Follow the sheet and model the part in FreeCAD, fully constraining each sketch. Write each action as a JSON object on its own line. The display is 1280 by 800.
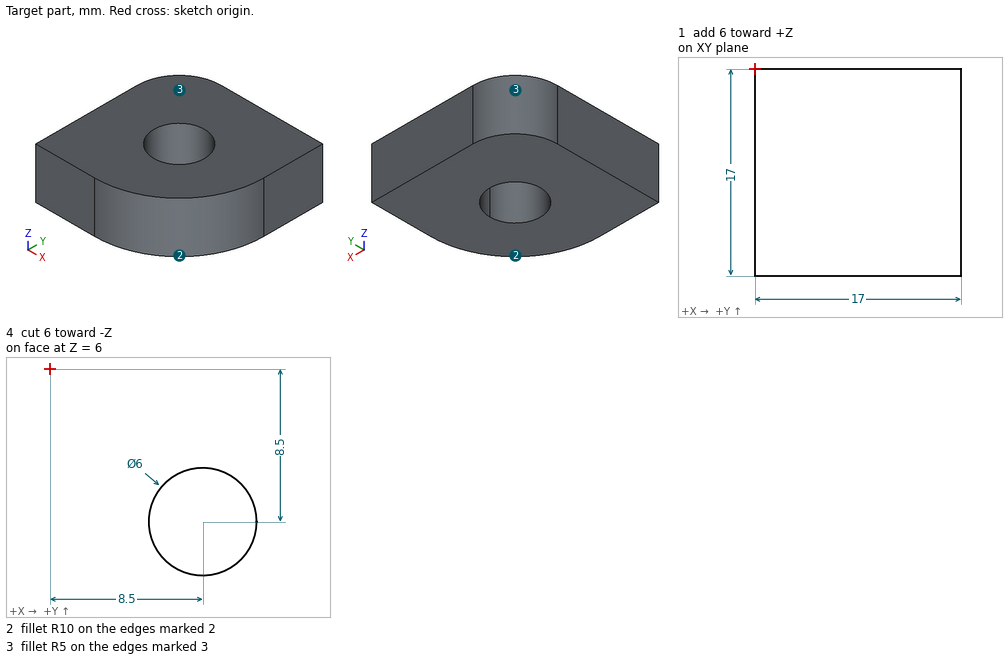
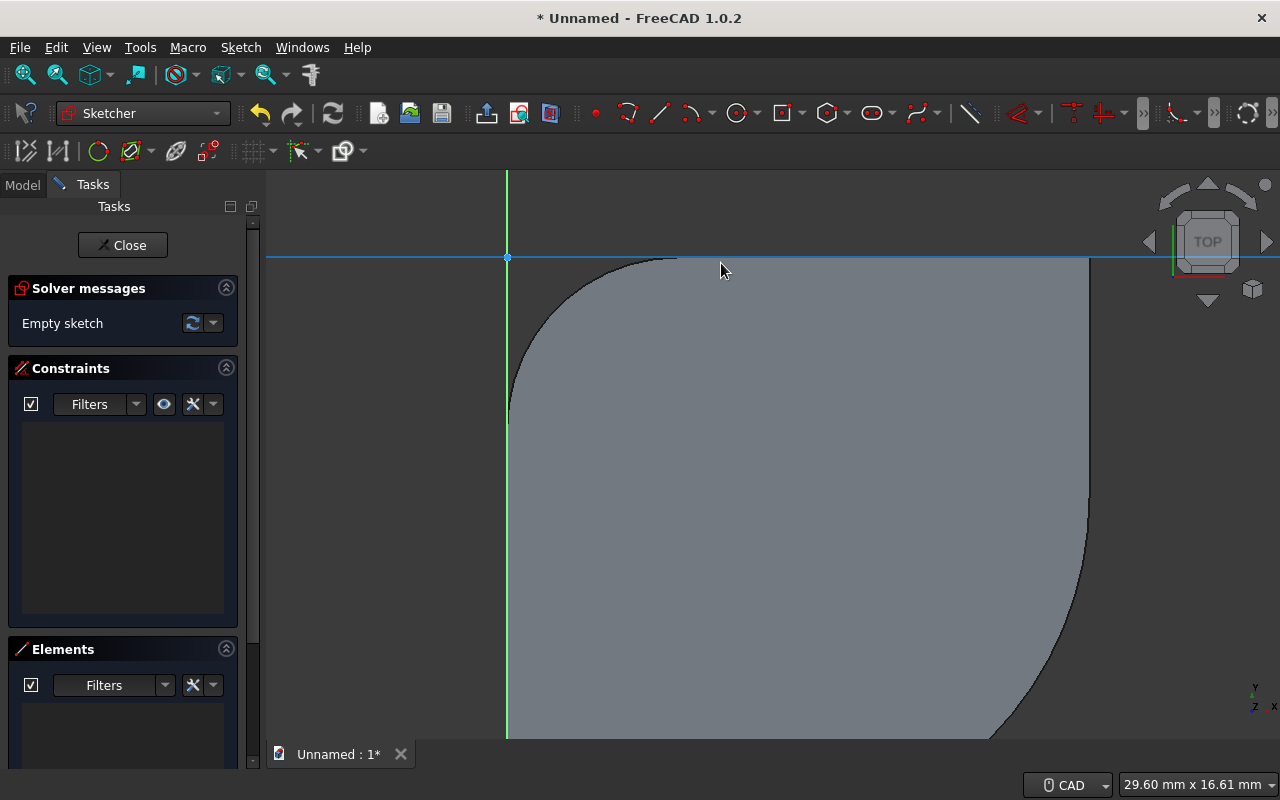
{"action": "left_click", "coordinate": [738, 114]}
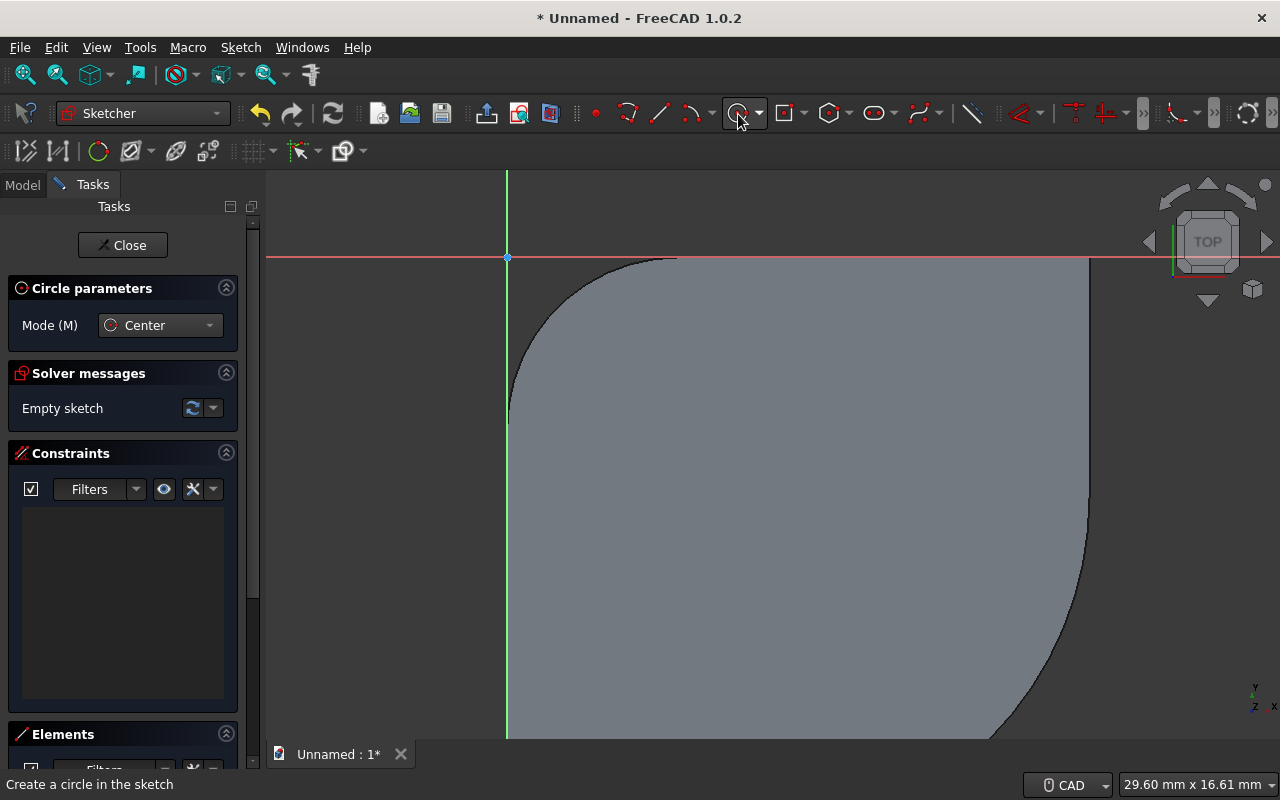
{"action": "left_click", "coordinate": [798, 549]}
{"action": "left_click", "coordinate": [871, 476]}
{"action": "key", "text": "Escape"}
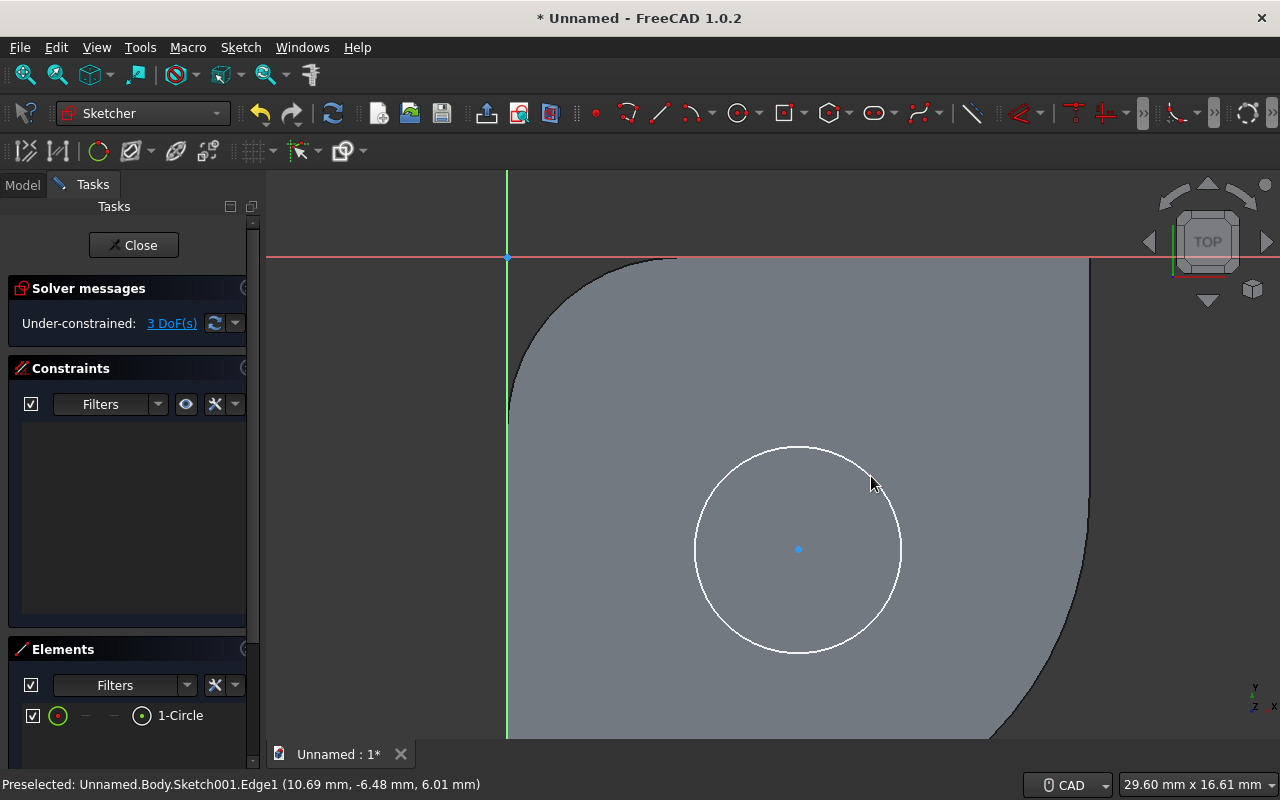
{"action": "left_click", "coordinate": [871, 477]}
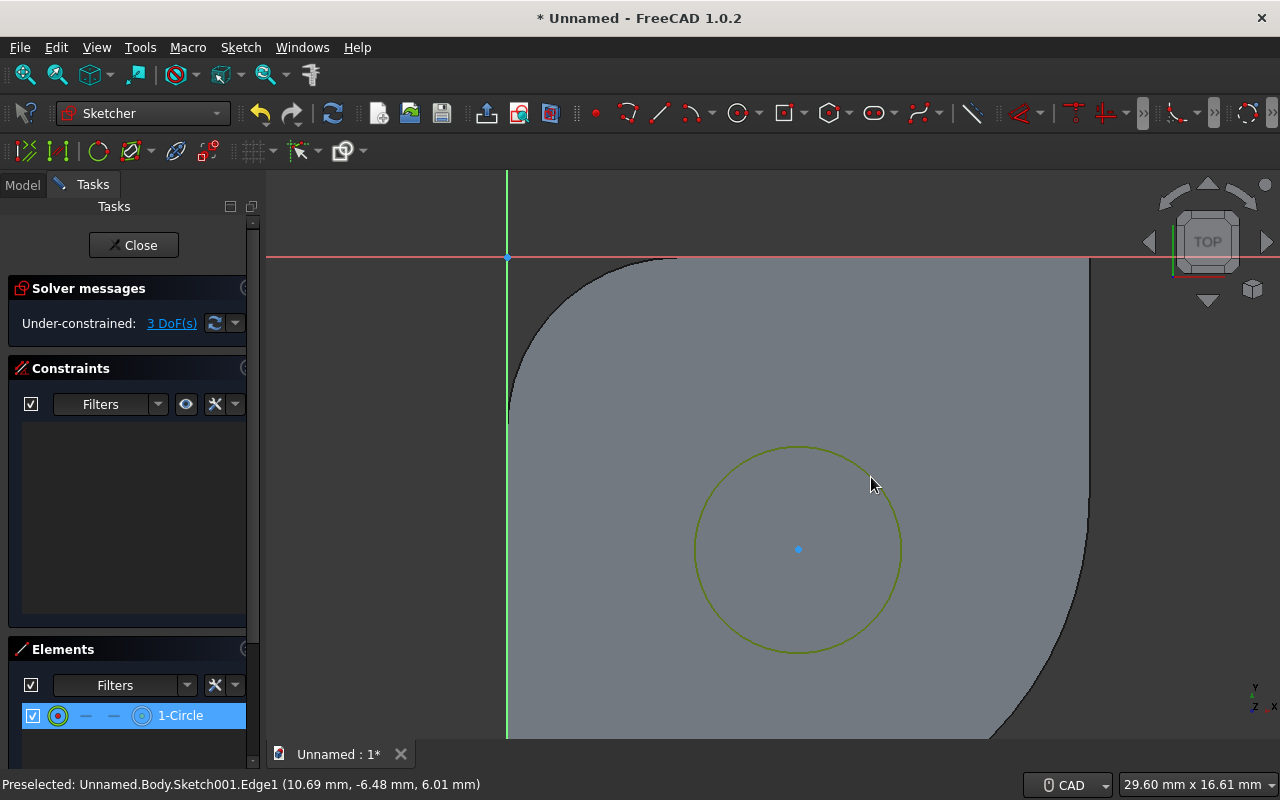
{"action": "left_click", "coordinate": [1042, 114]}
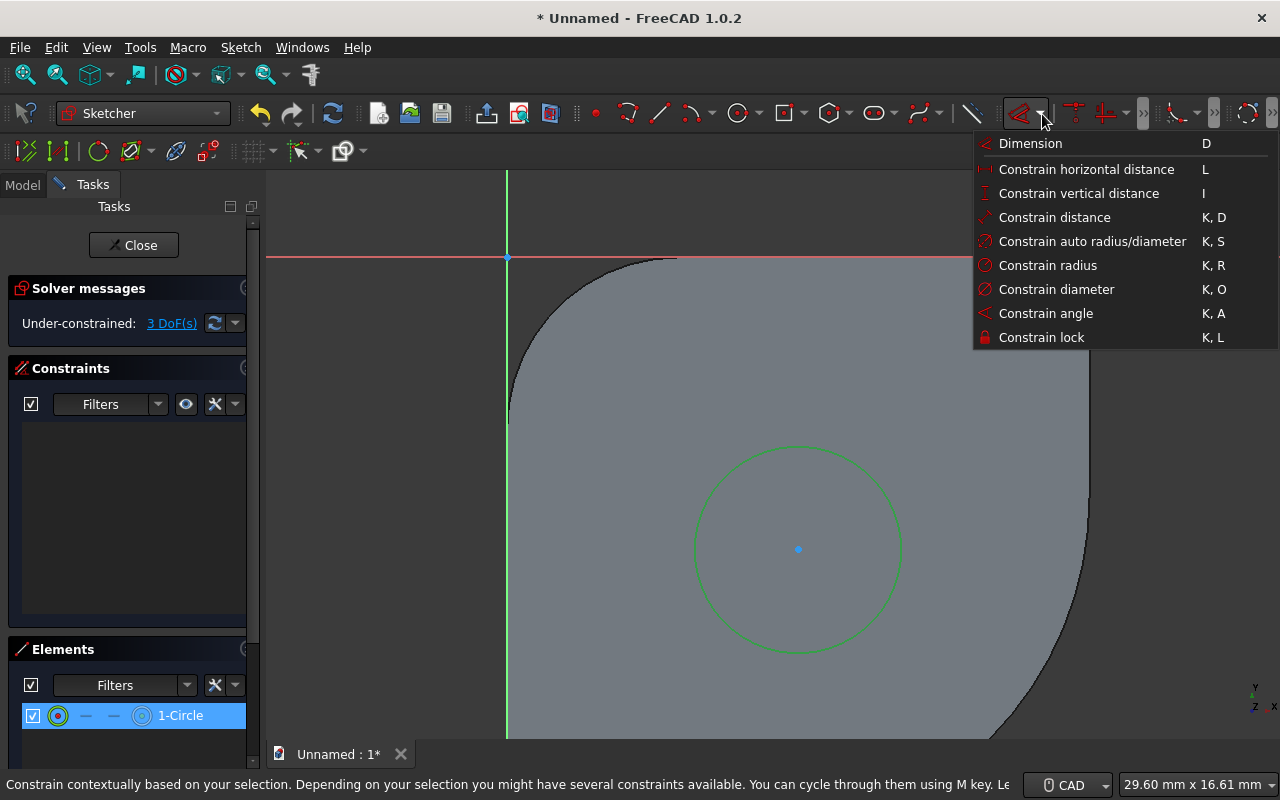
{"action": "left_click", "coordinate": [1126, 289]}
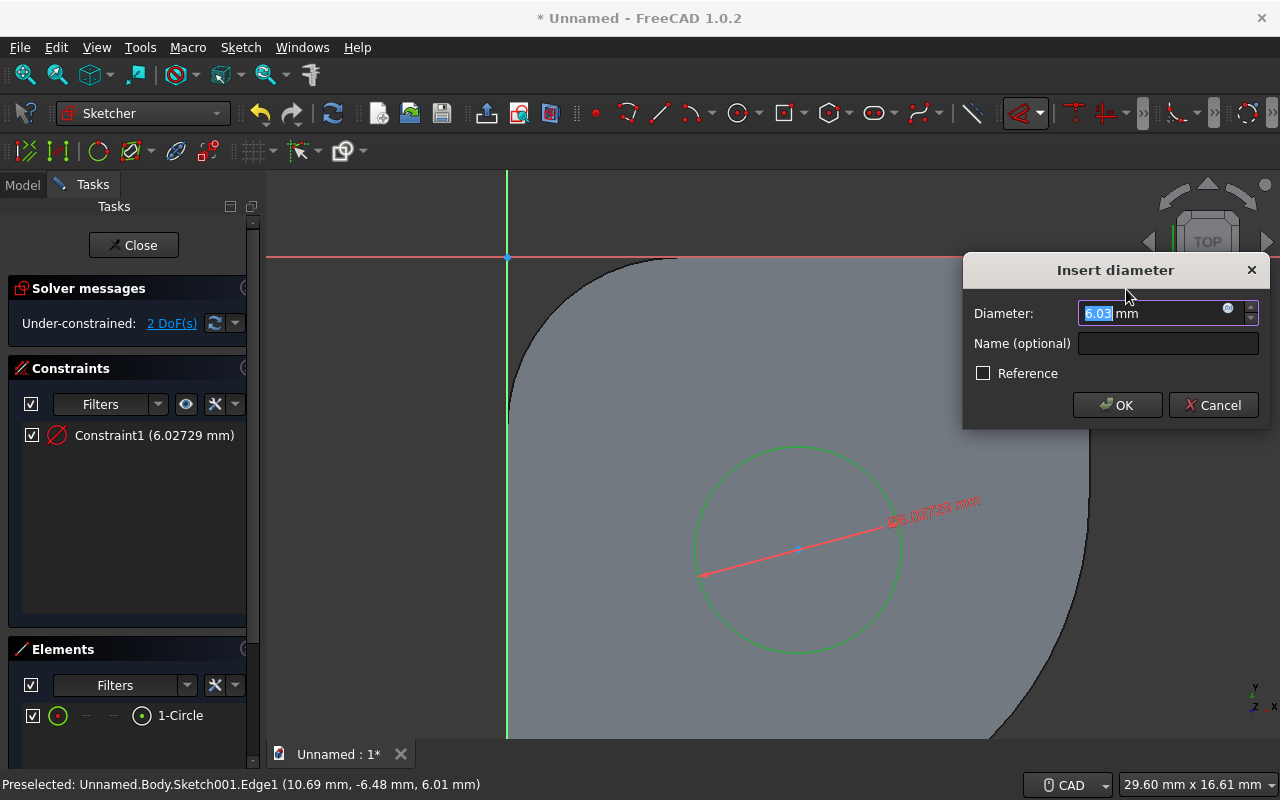
{"action": "type", "text": "6"}
{"action": "key", "text": "Return"}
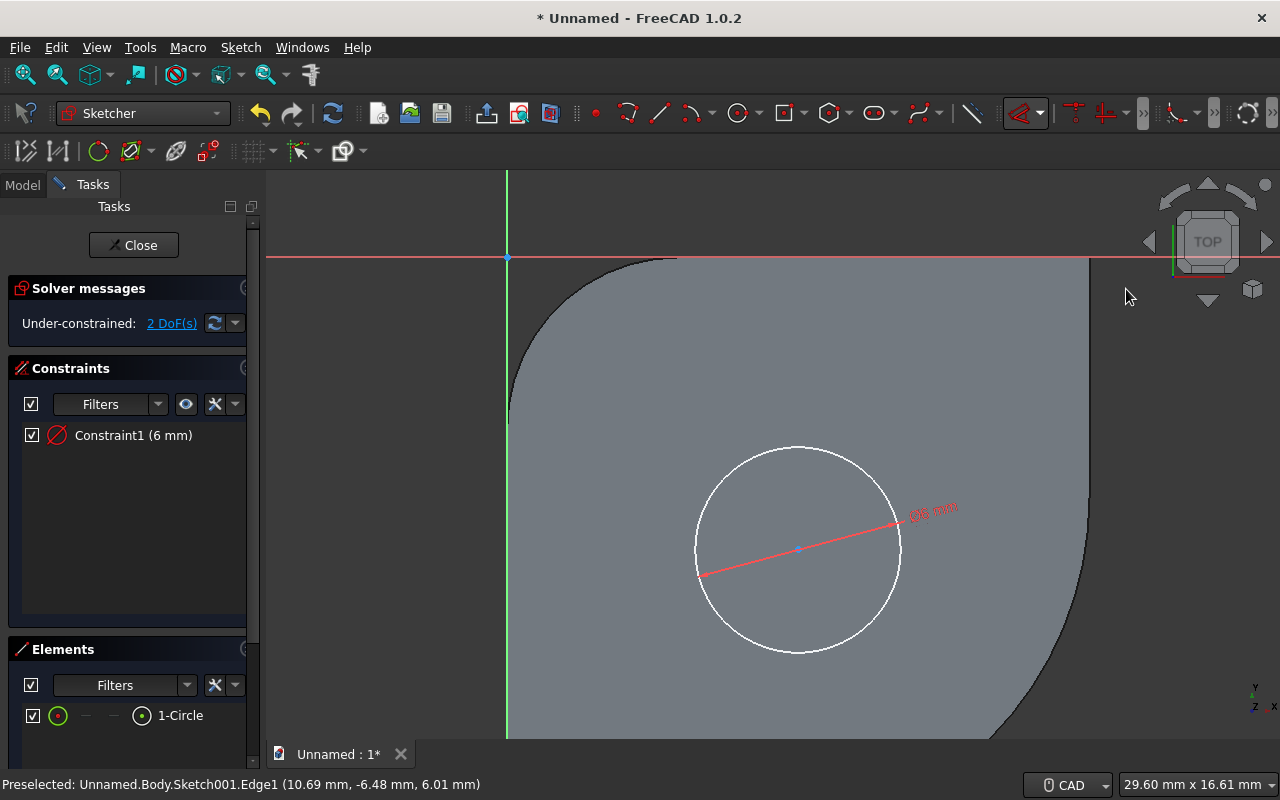
{"action": "left_click", "coordinate": [798, 550]}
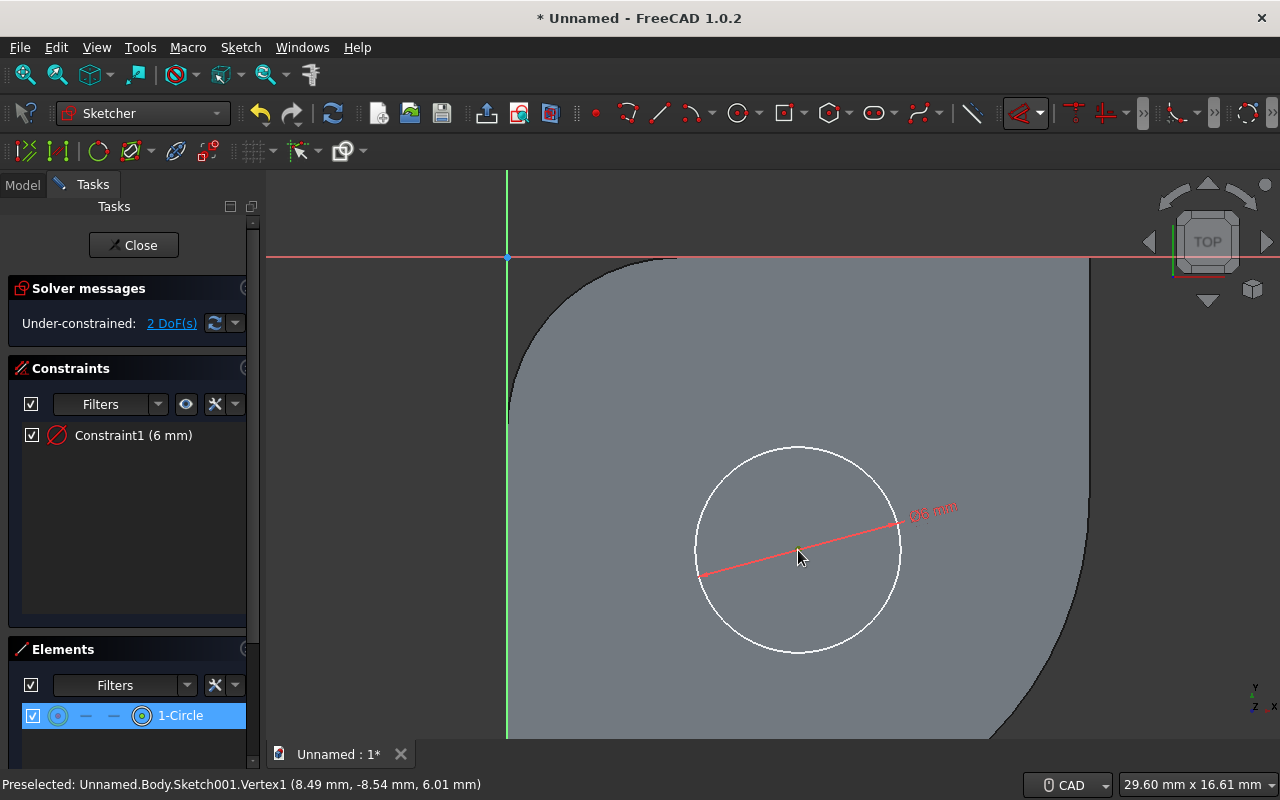
{"action": "key", "text": "l"}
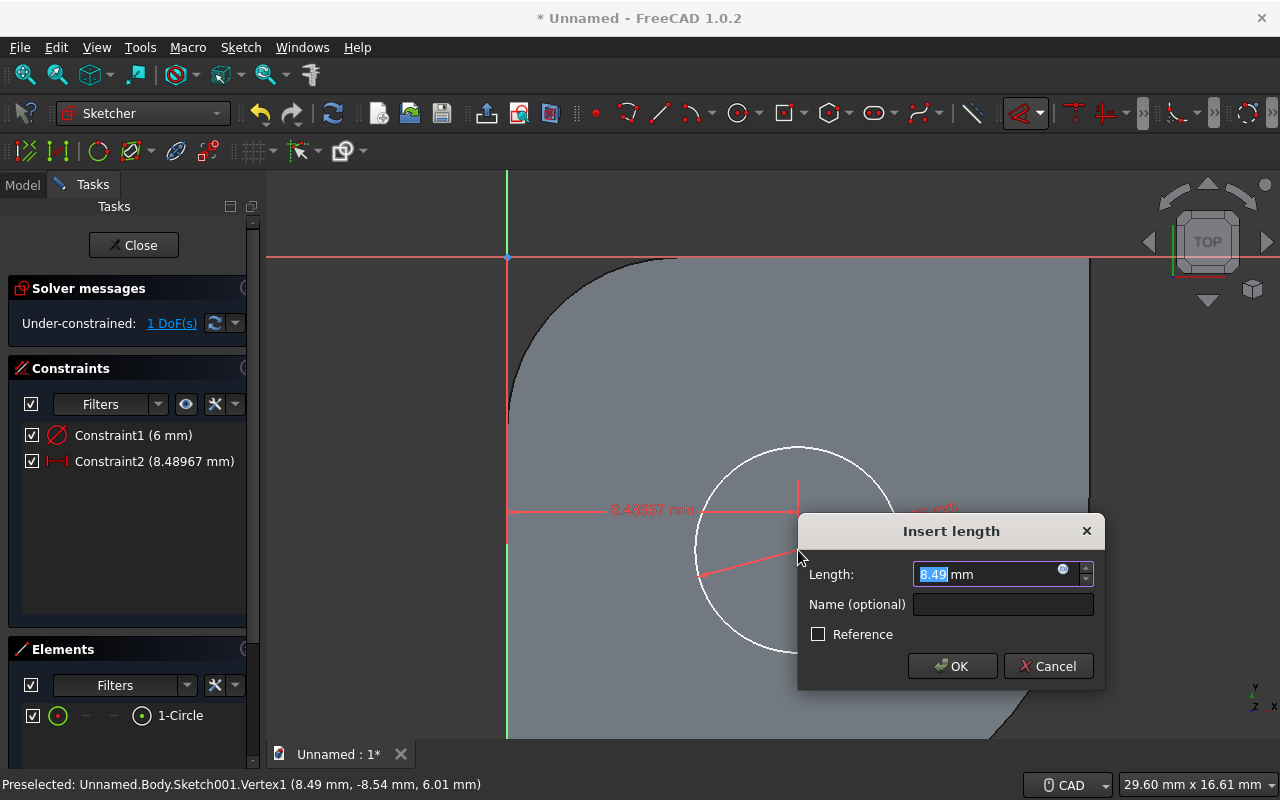
{"action": "type", "text": "8.5"}
{"action": "key", "text": "Return"}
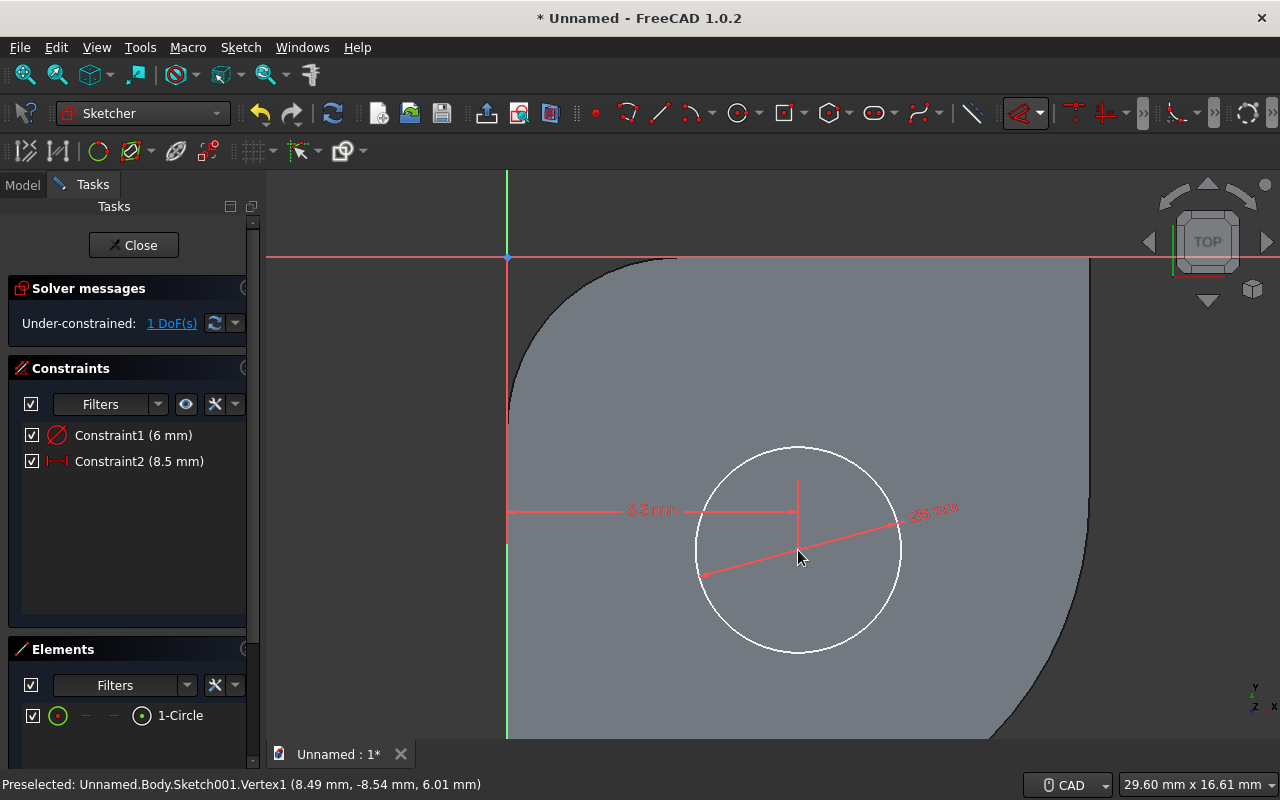
{"action": "left_click", "coordinate": [798, 550]}